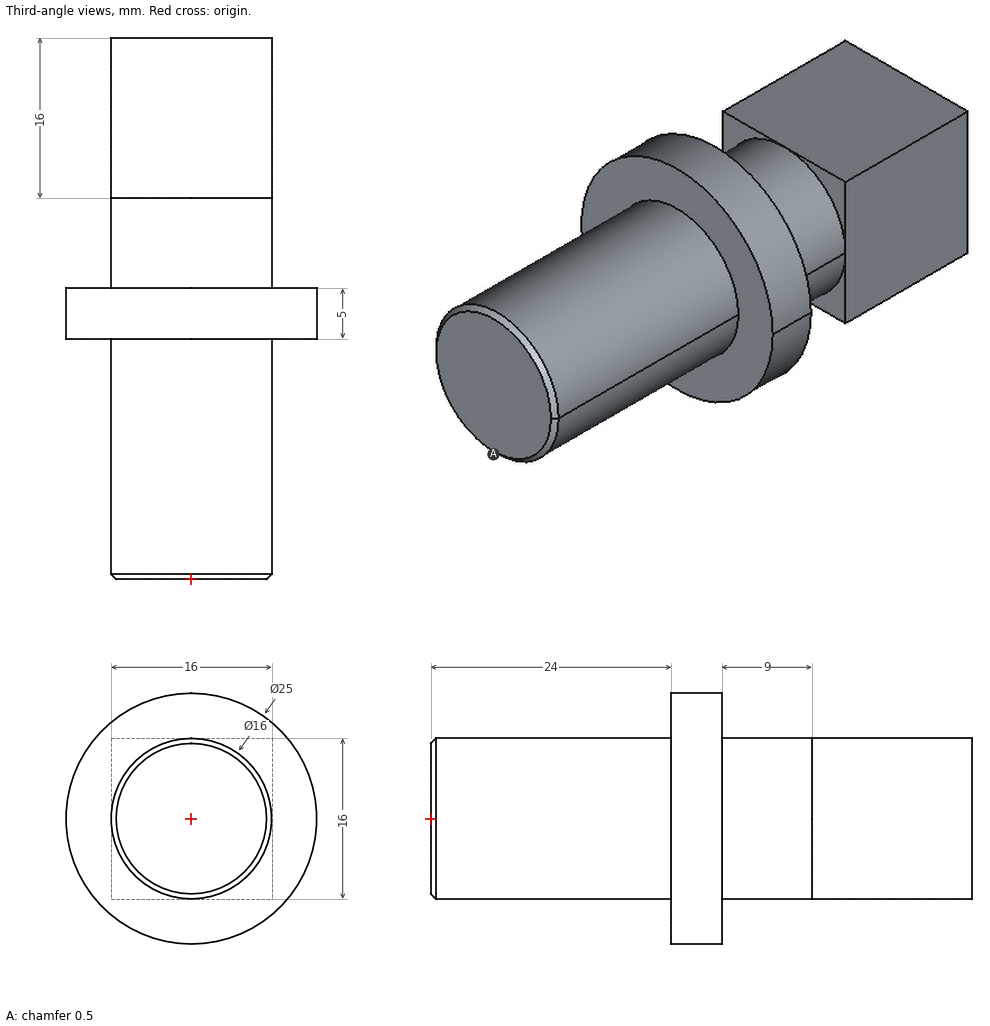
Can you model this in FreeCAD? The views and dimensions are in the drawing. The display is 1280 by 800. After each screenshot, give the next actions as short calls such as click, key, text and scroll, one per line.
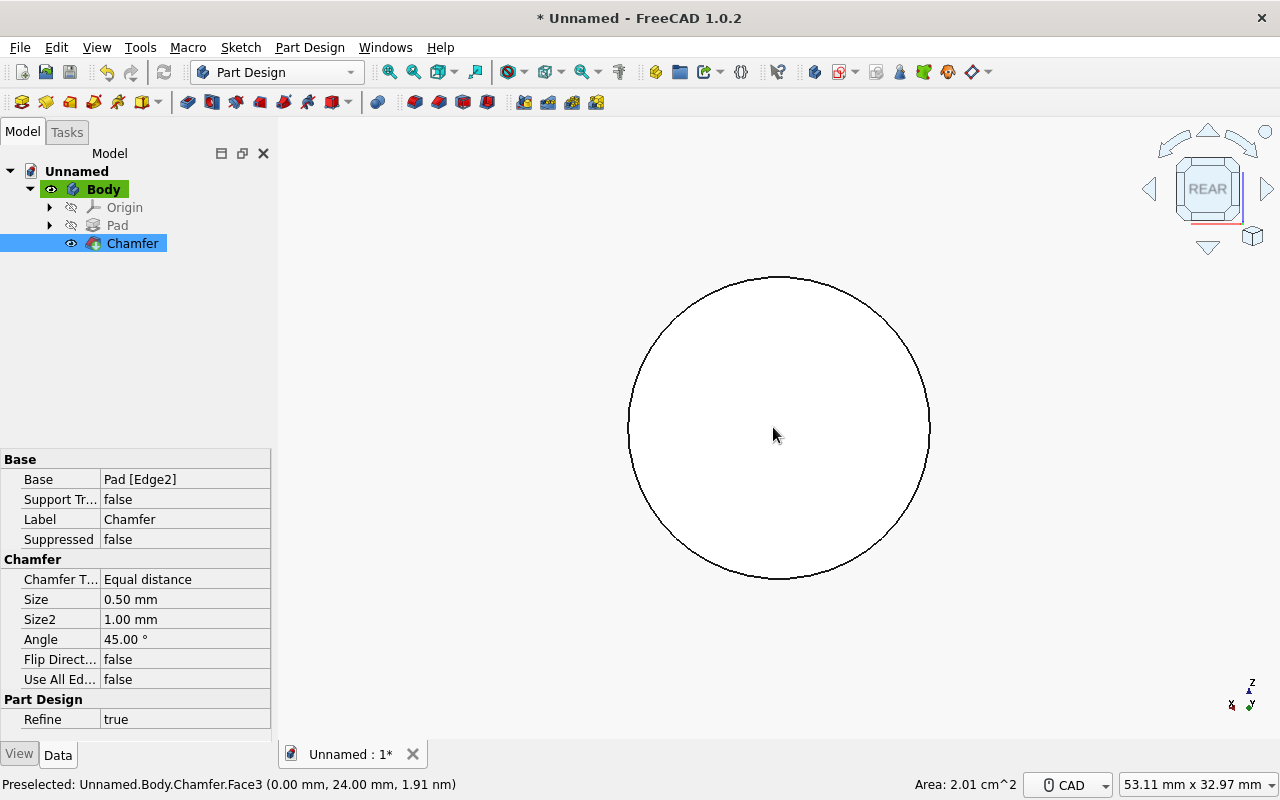
click(840, 72)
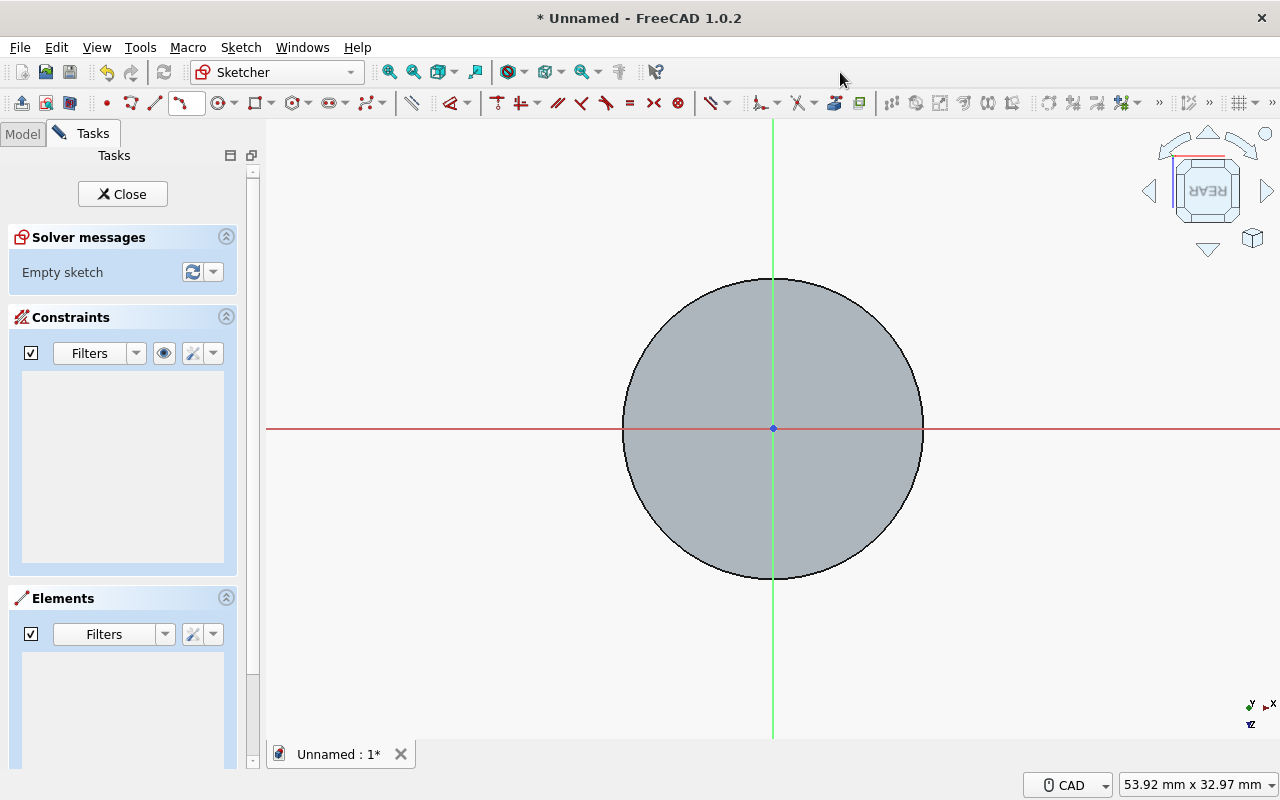
click(218, 104)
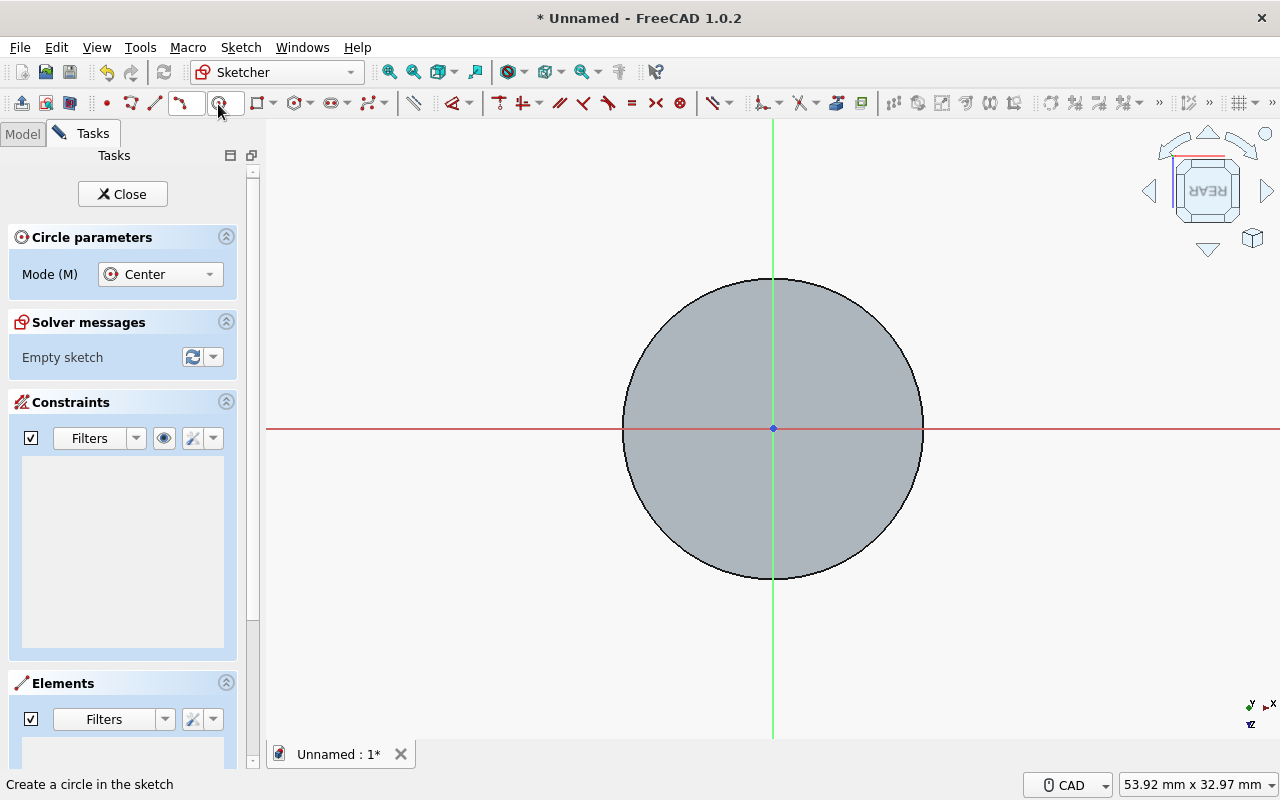
click(773, 429)
move(939, 263)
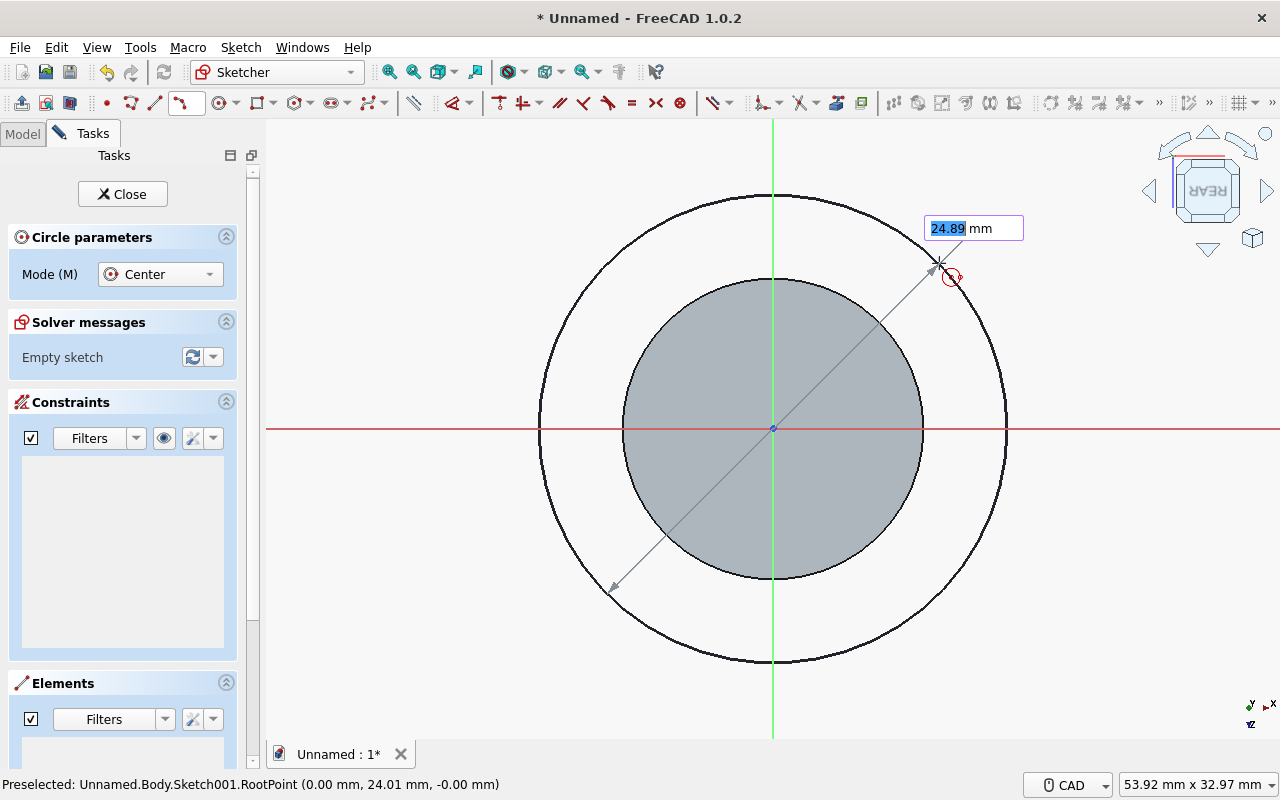
text(25)
key(Return)
key(Escape)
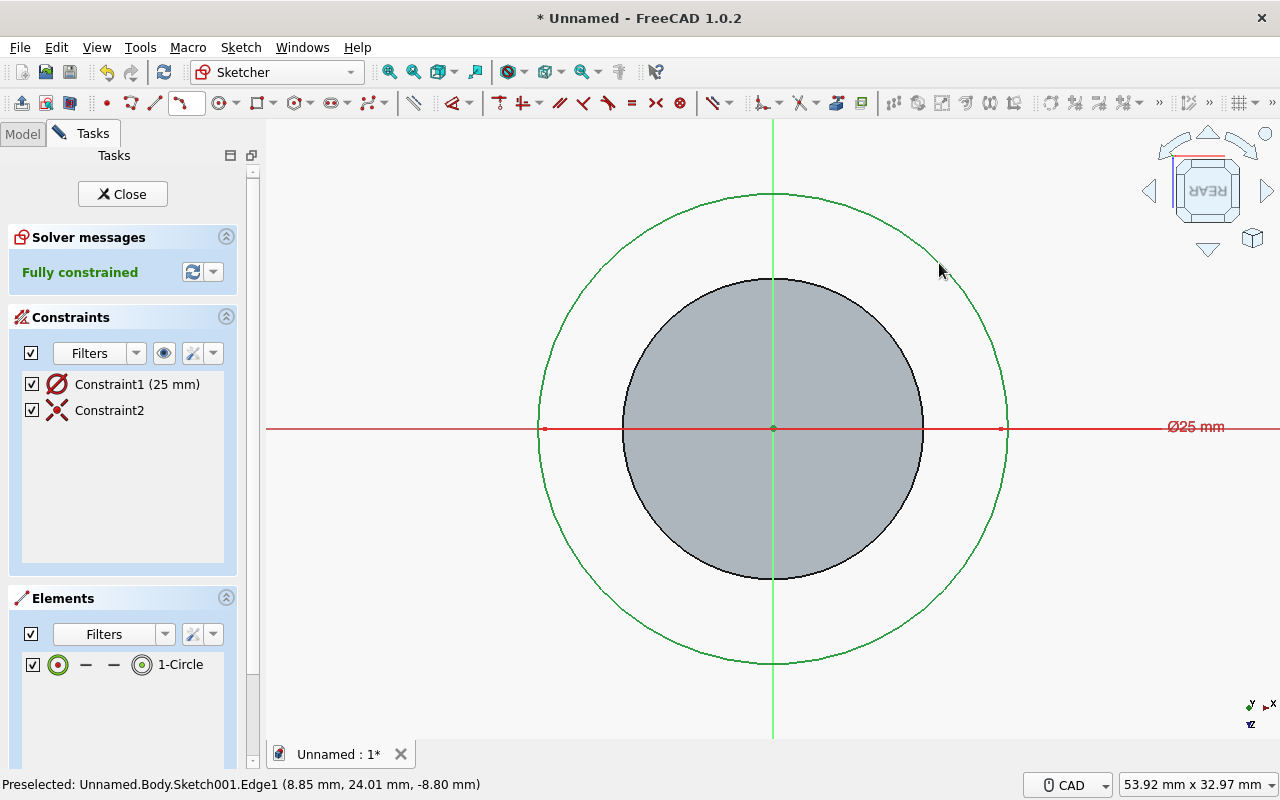
click(123, 194)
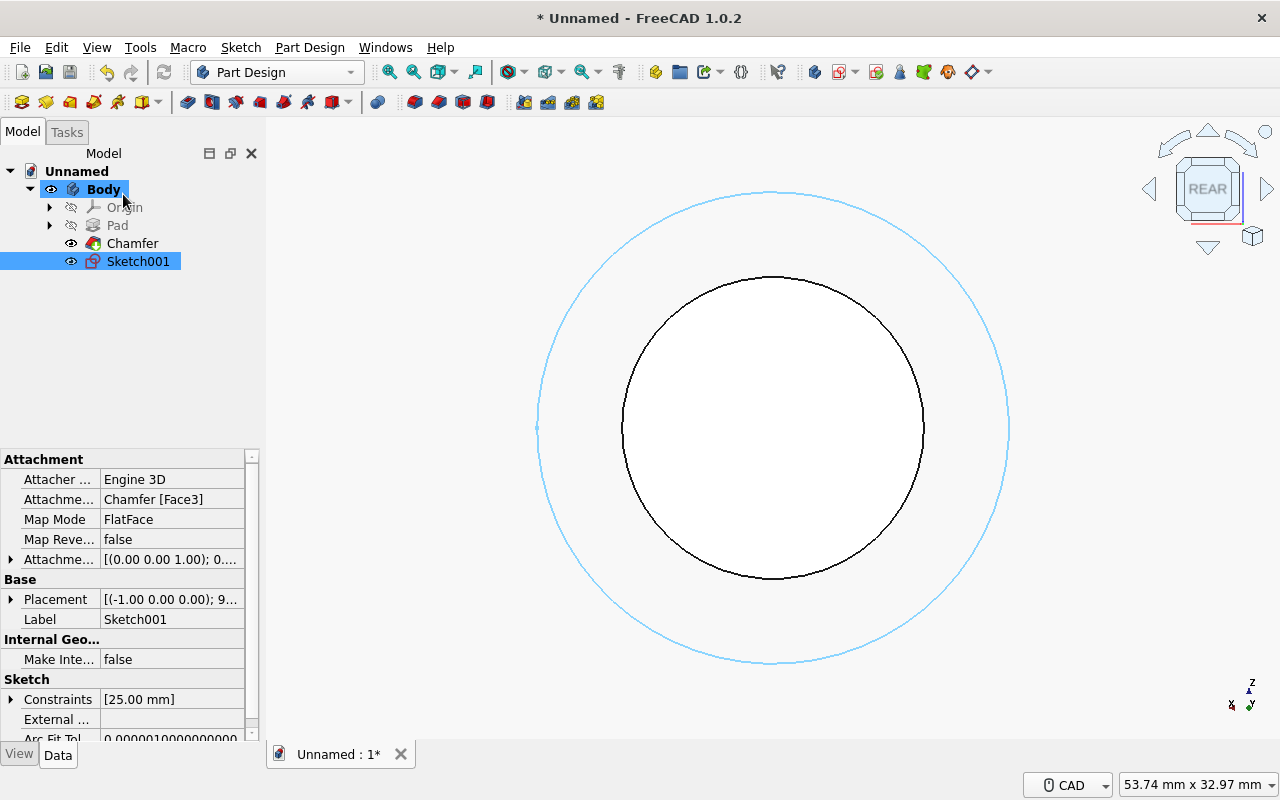
click(22, 102)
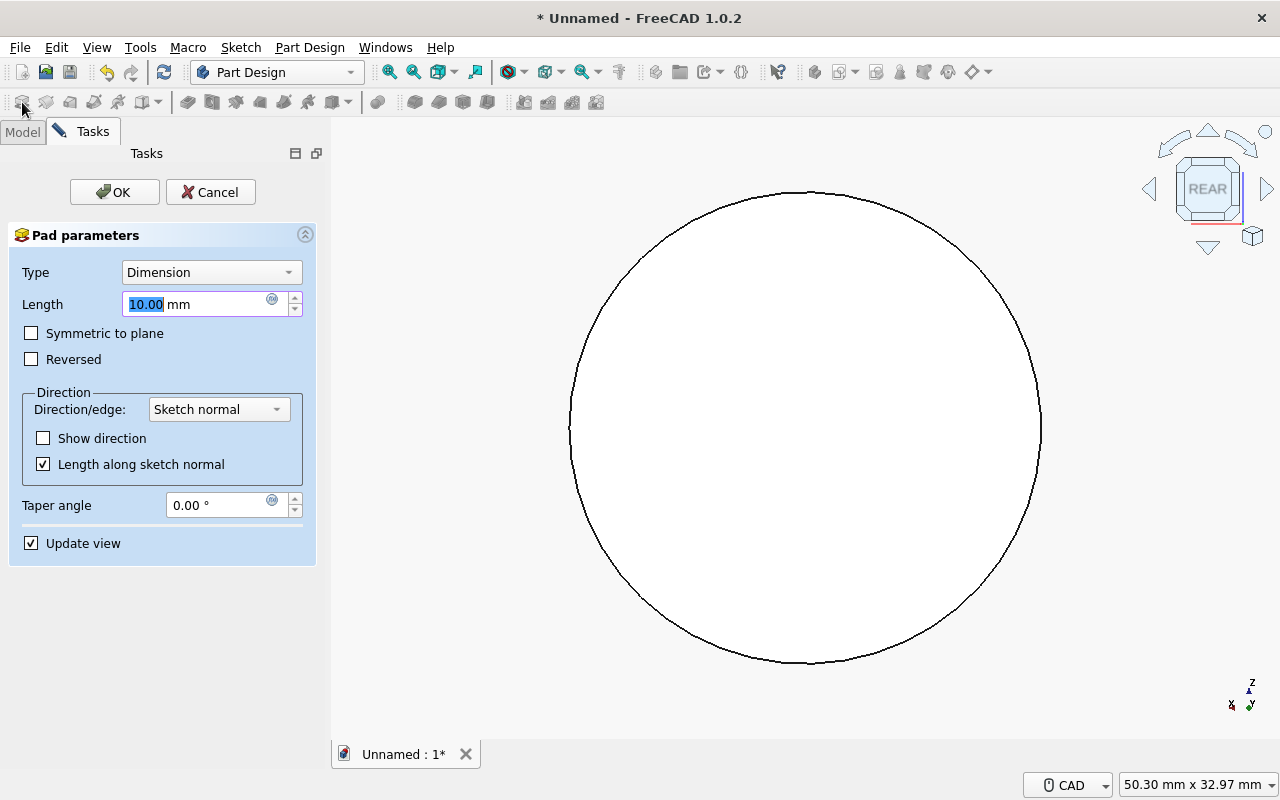
text(5)
key(Tab)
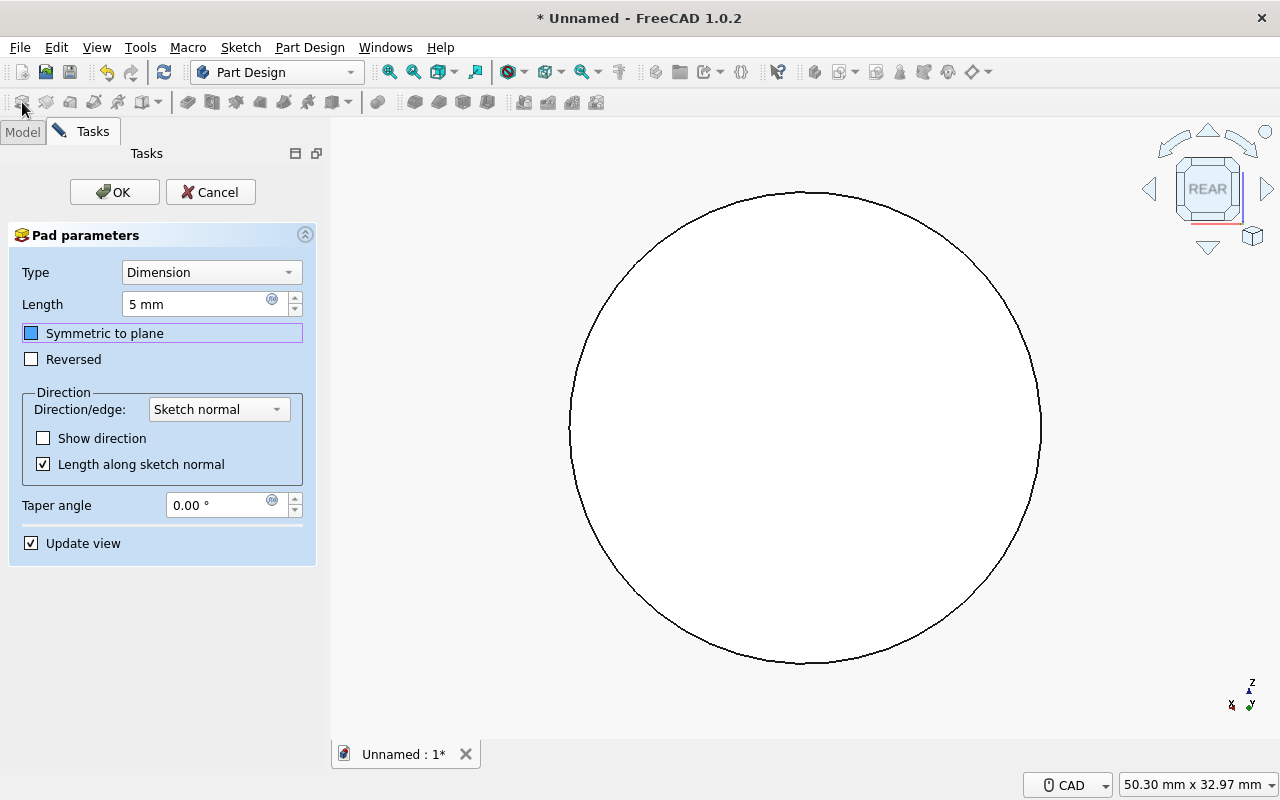
click(115, 192)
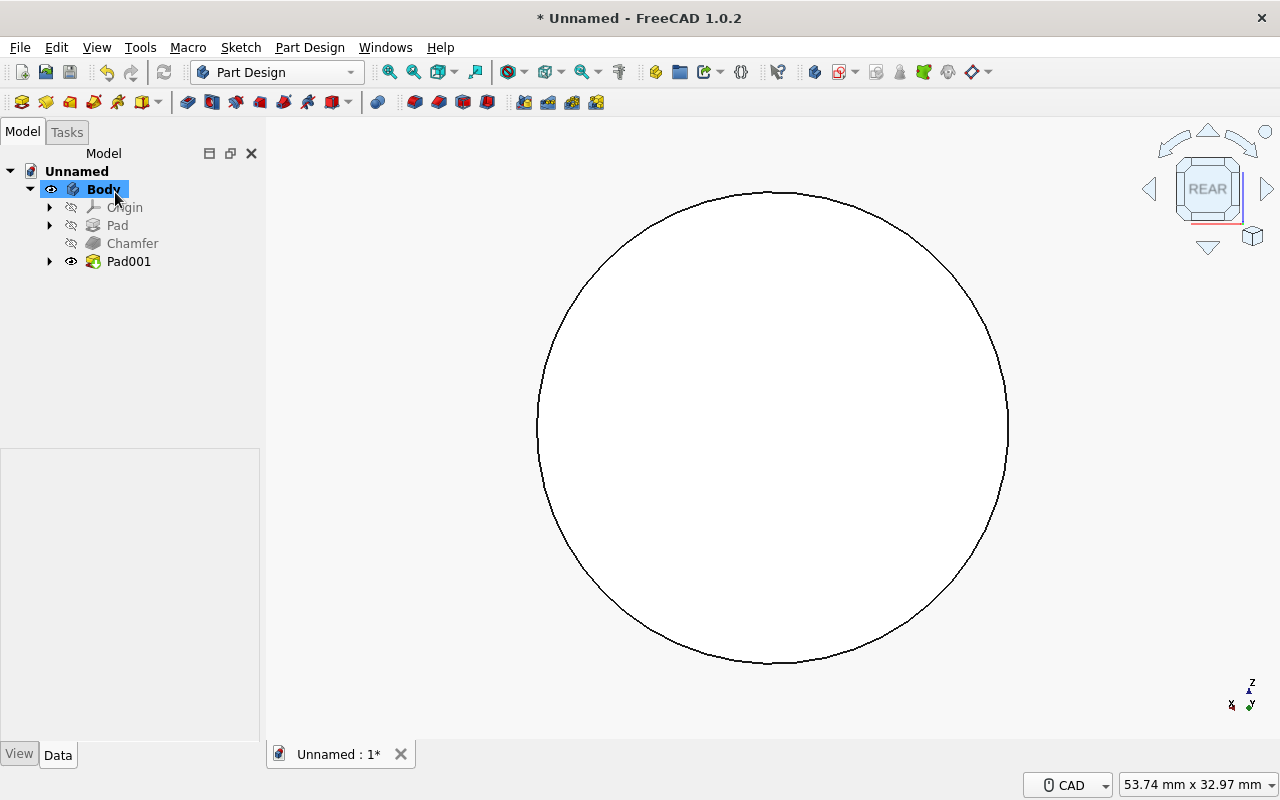
click(773, 427)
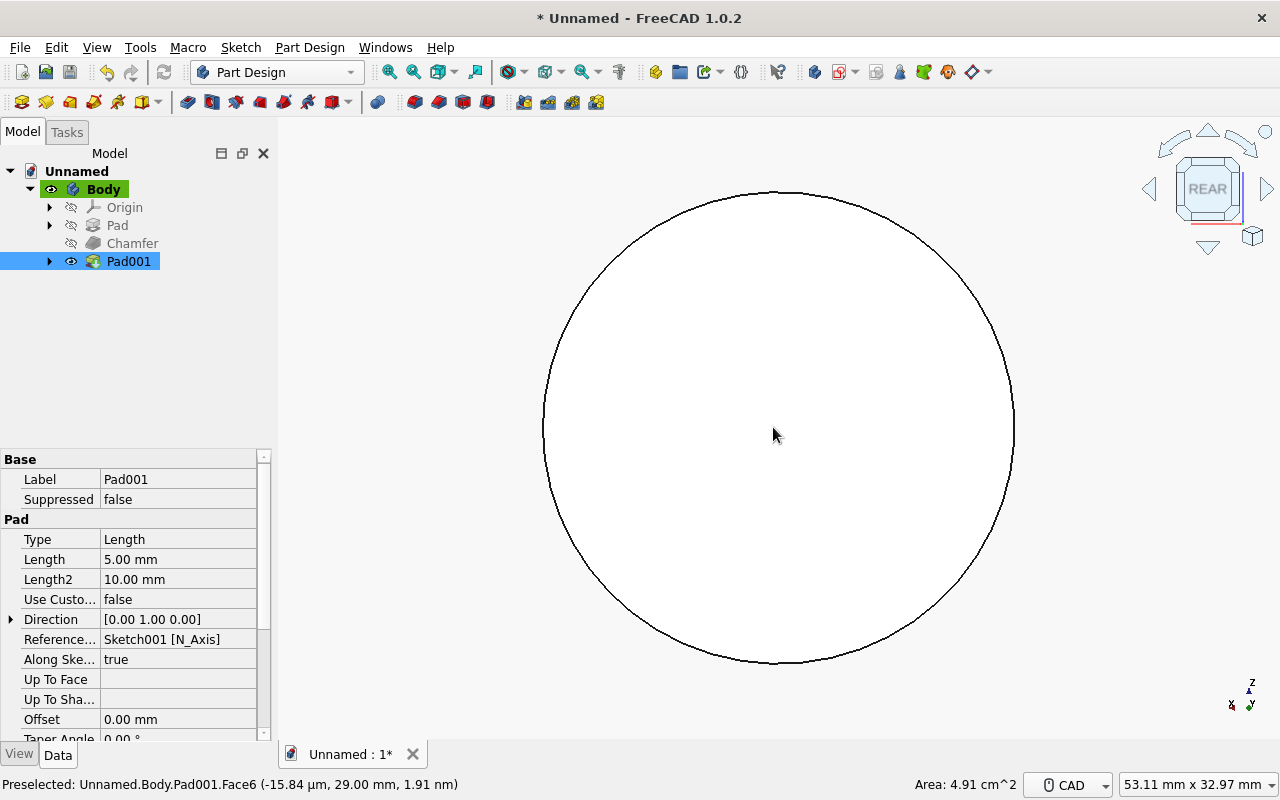
click(840, 72)